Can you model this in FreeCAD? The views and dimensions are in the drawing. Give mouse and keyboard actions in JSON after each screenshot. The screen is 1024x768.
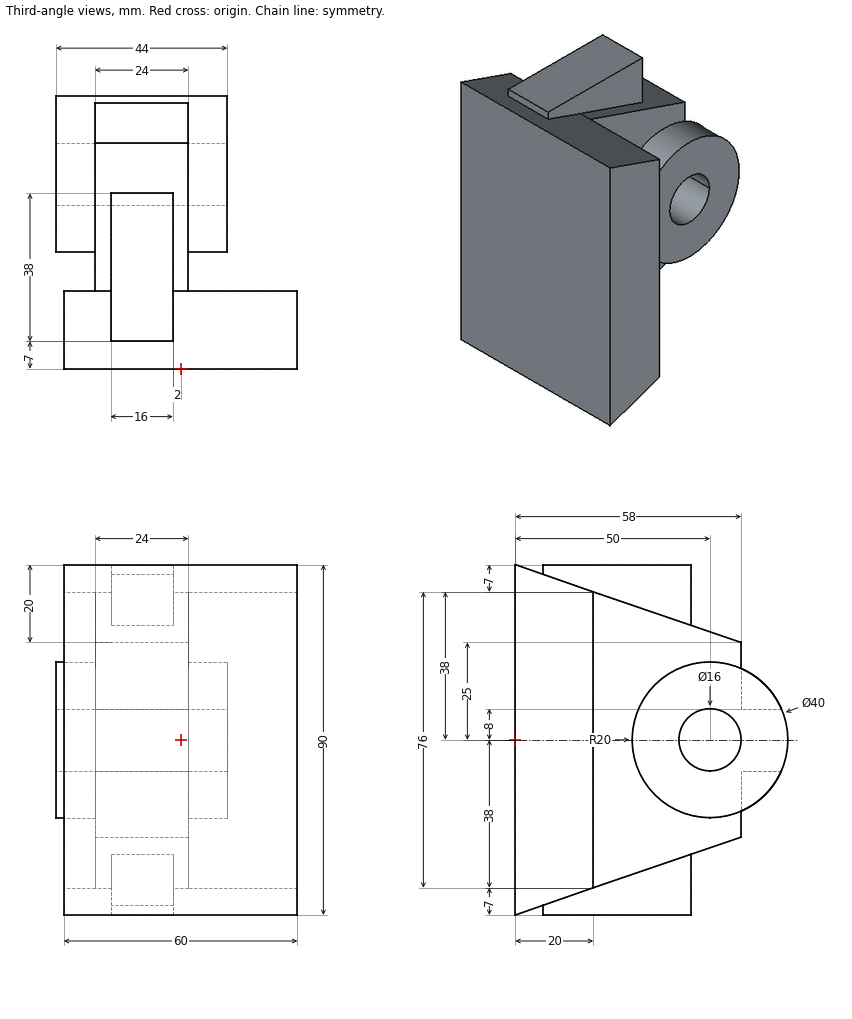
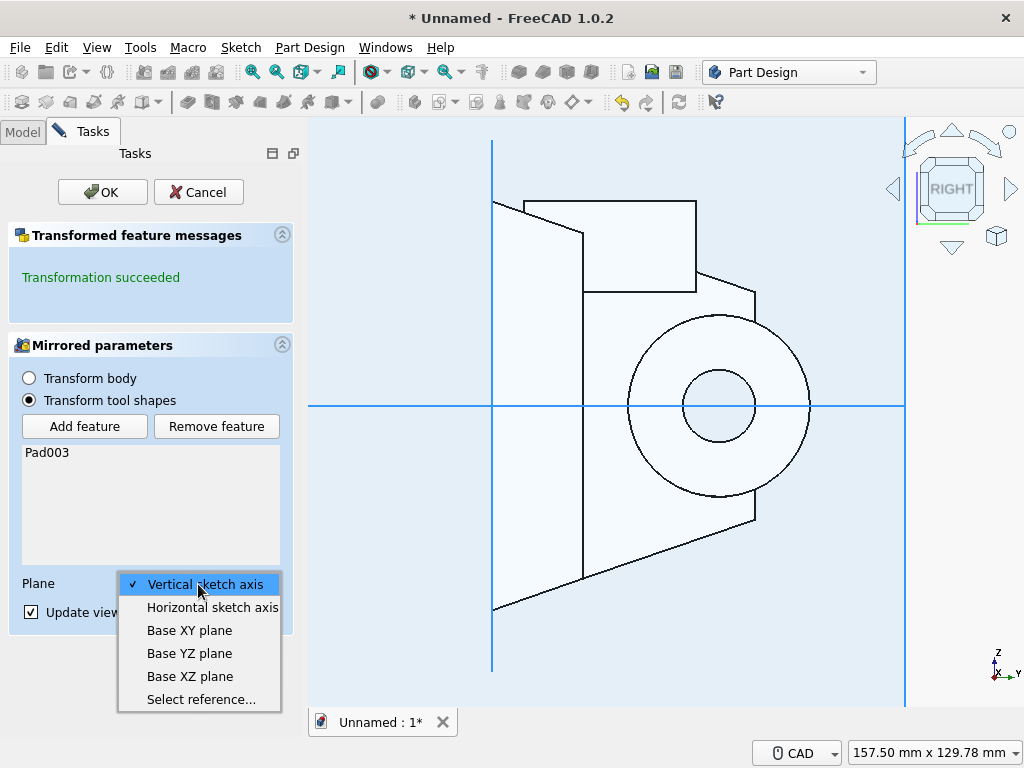
{"action": "left_click", "coordinate": [198, 630]}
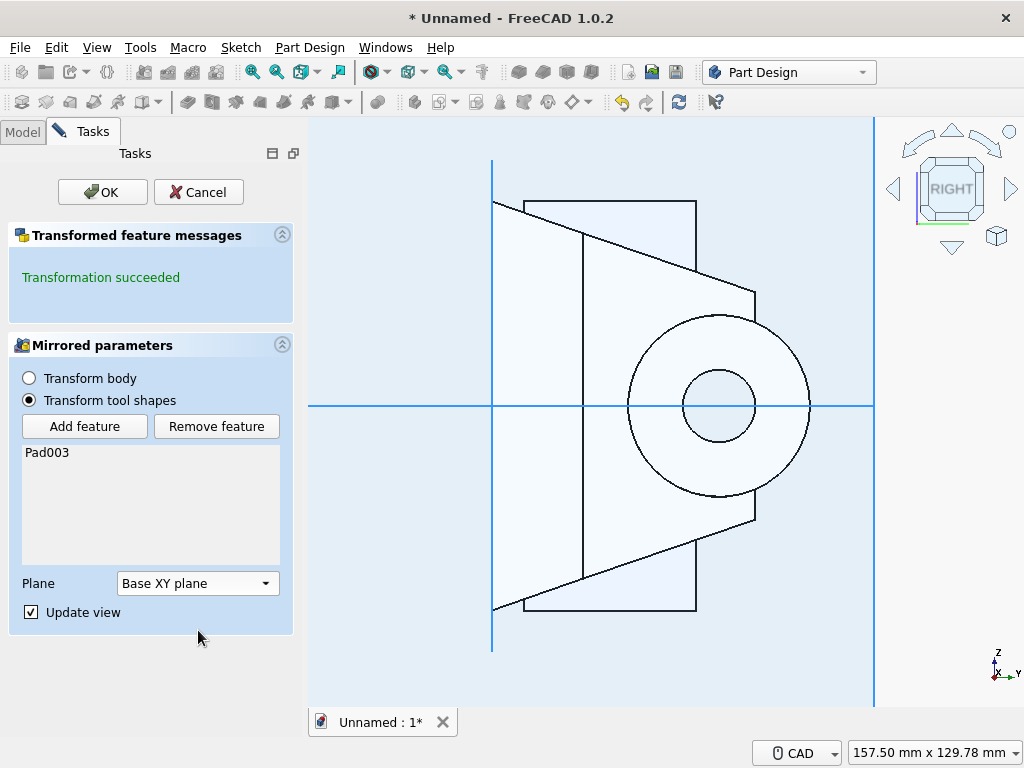
{"action": "left_click", "coordinate": [103, 192]}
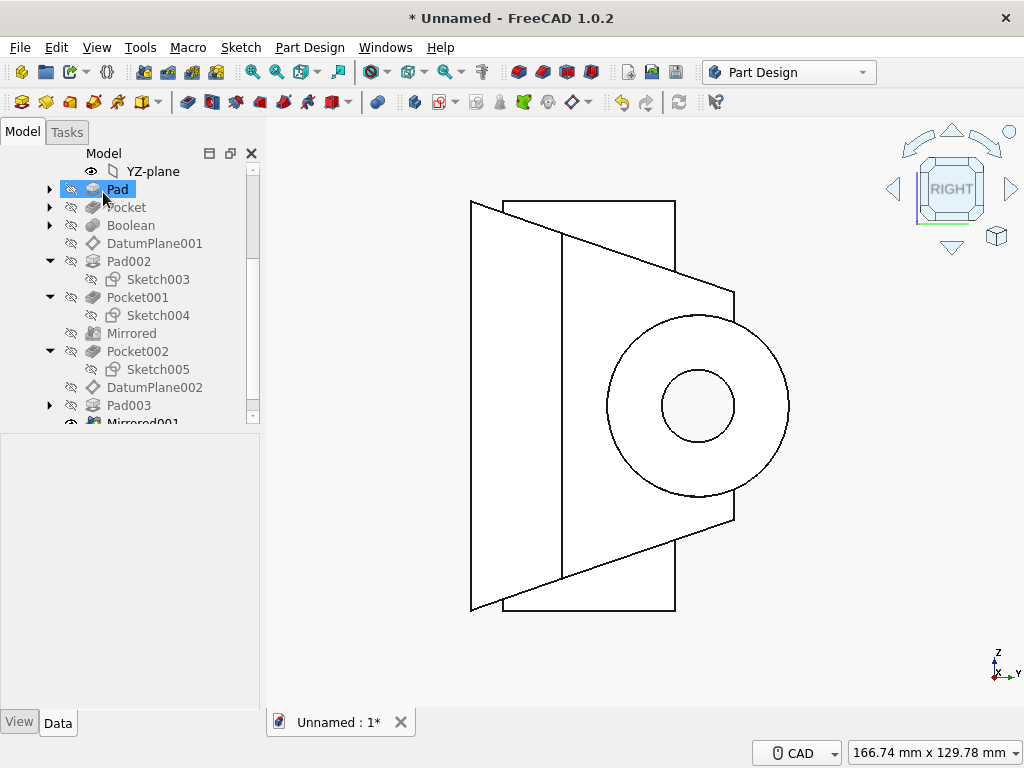
{"action": "key", "text": "0"}